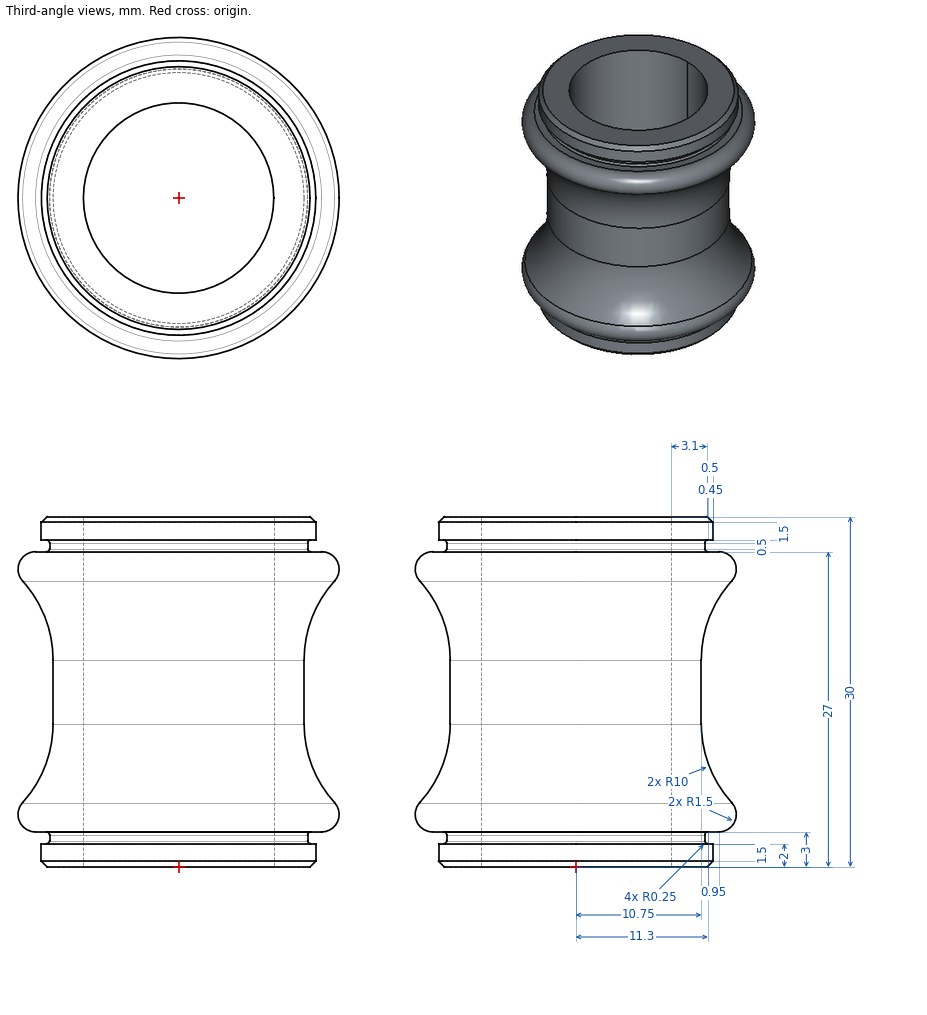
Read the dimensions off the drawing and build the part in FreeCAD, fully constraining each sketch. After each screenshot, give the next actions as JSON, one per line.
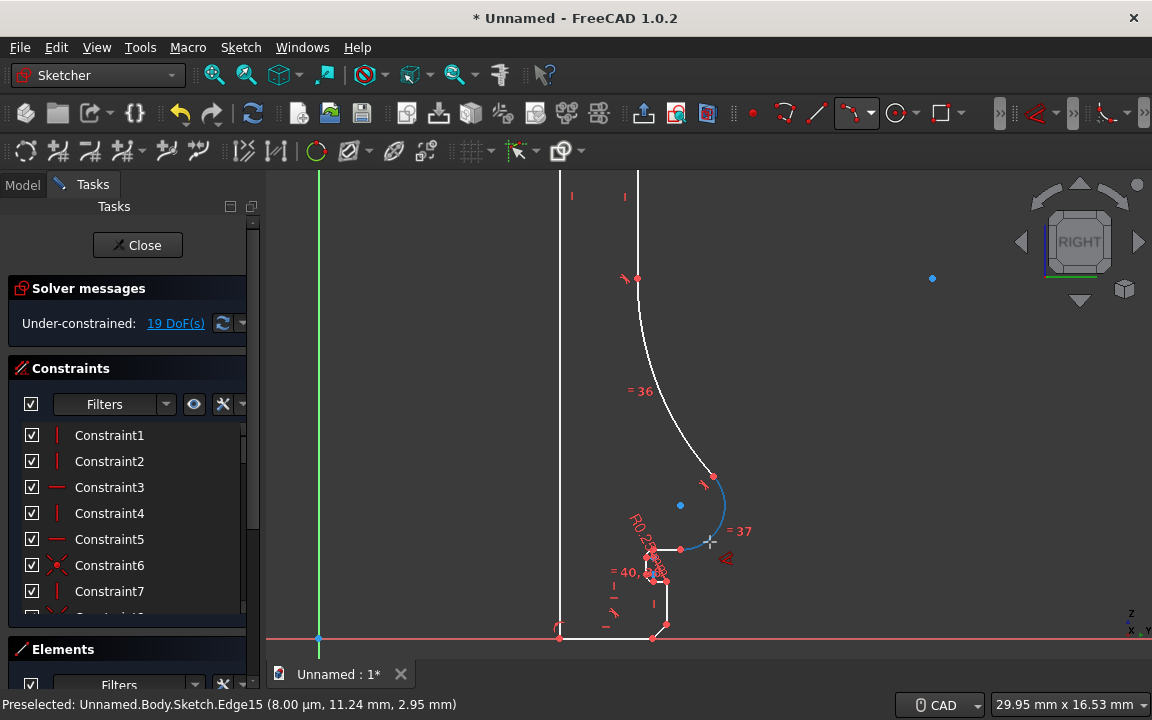
{"action": "left_click", "coordinate": [709, 540]}
{"action": "left_click", "coordinate": [729, 565]}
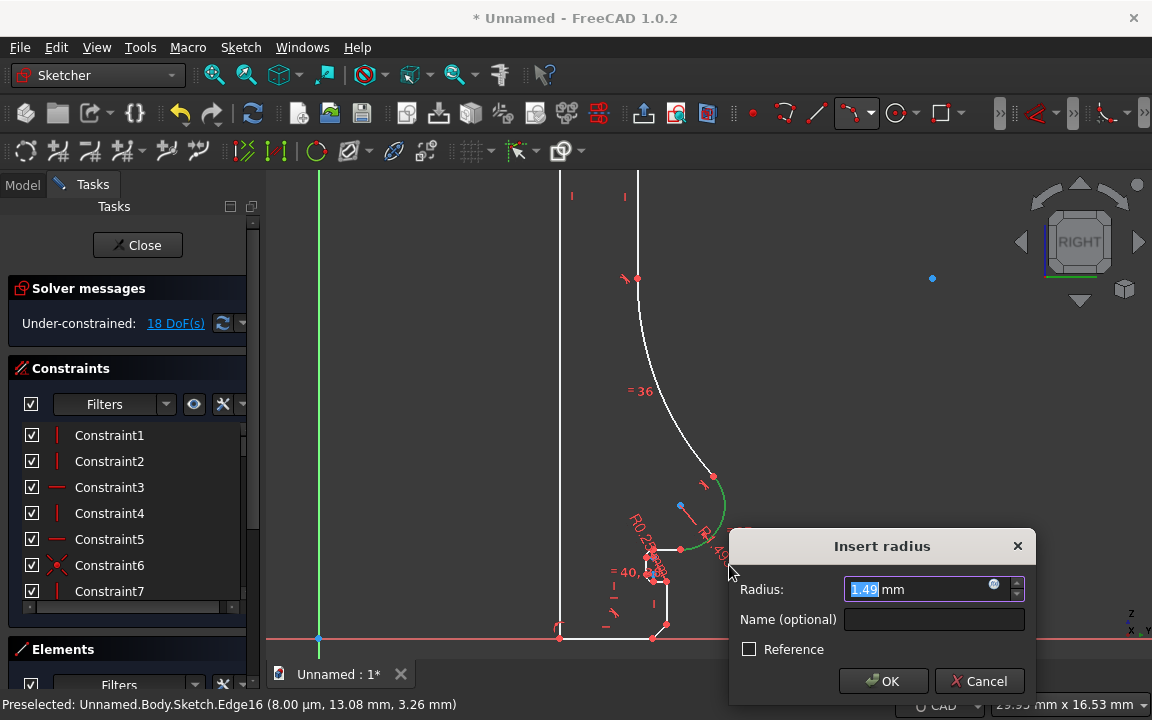
{"action": "type", "text": "1.5"}
{"action": "key", "text": "Return"}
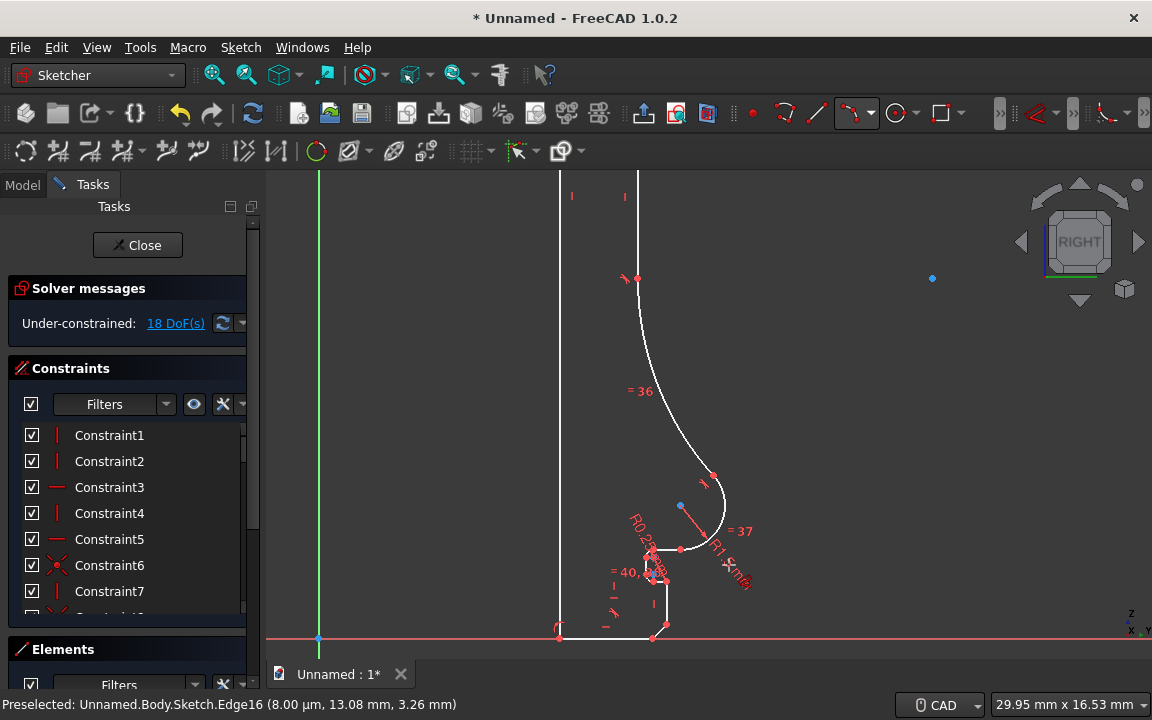
{"action": "left_click", "coordinate": [645, 343]}
{"action": "left_click", "coordinate": [614, 350]}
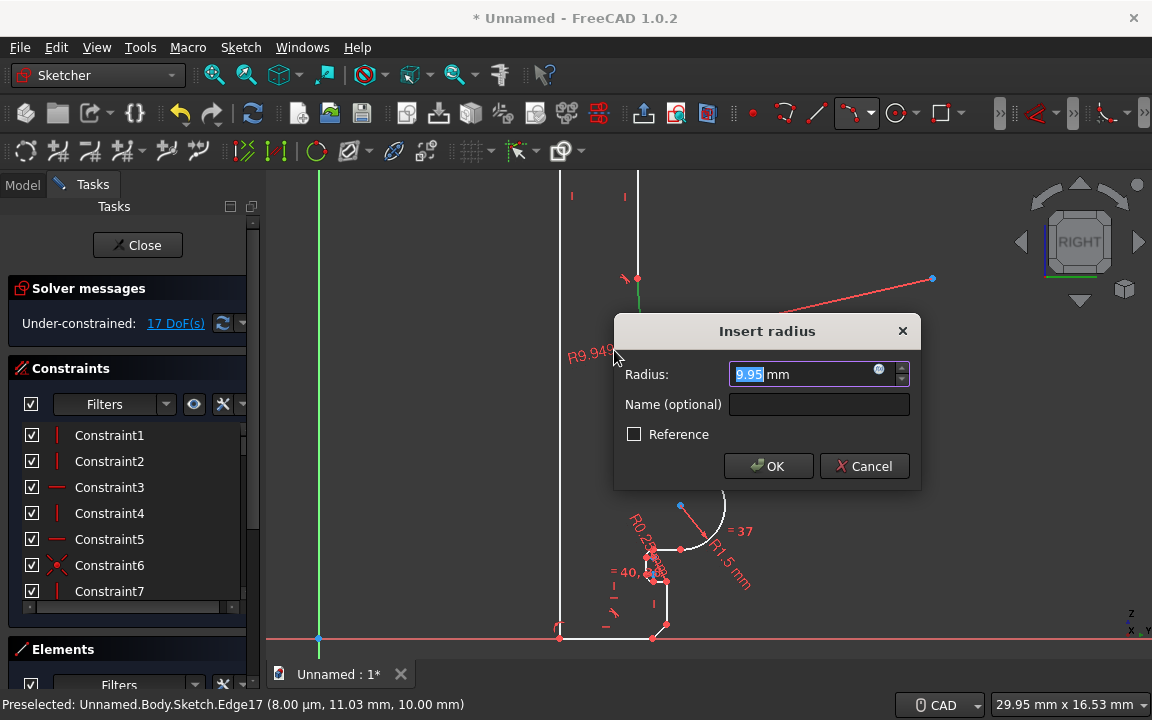
{"action": "type", "text": "10"}
{"action": "key", "text": "Return"}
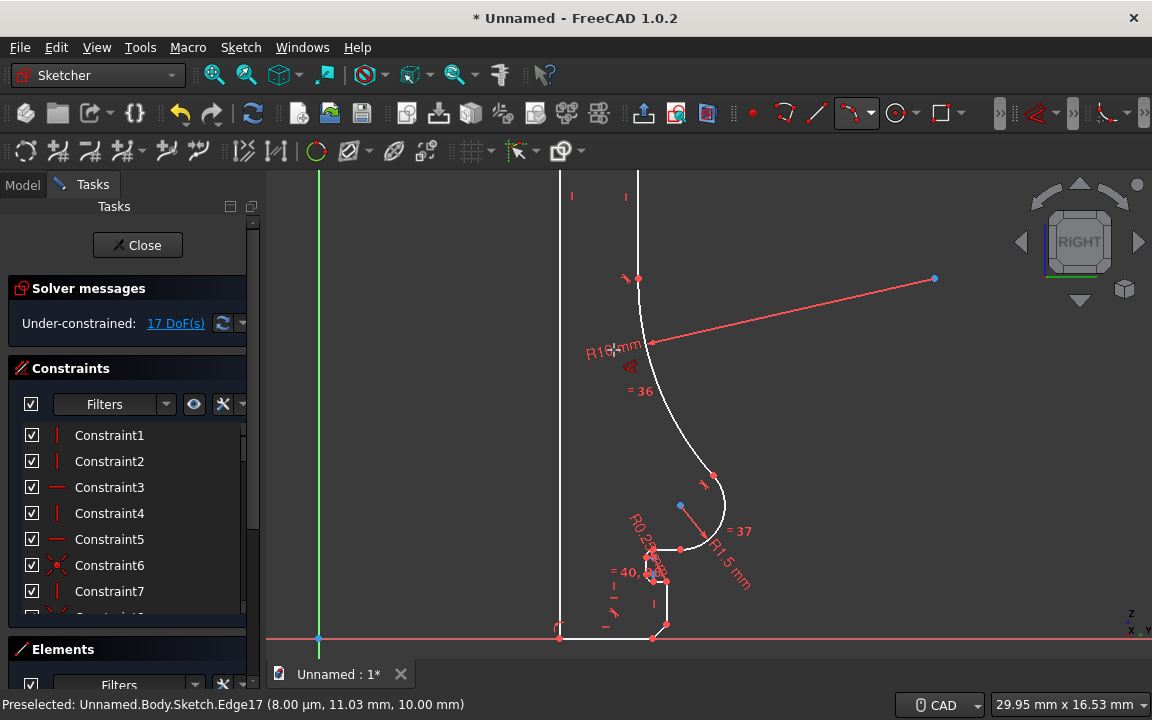
{"action": "left_click", "coordinate": [560, 373]}
{"action": "left_click", "coordinate": [594, 414]}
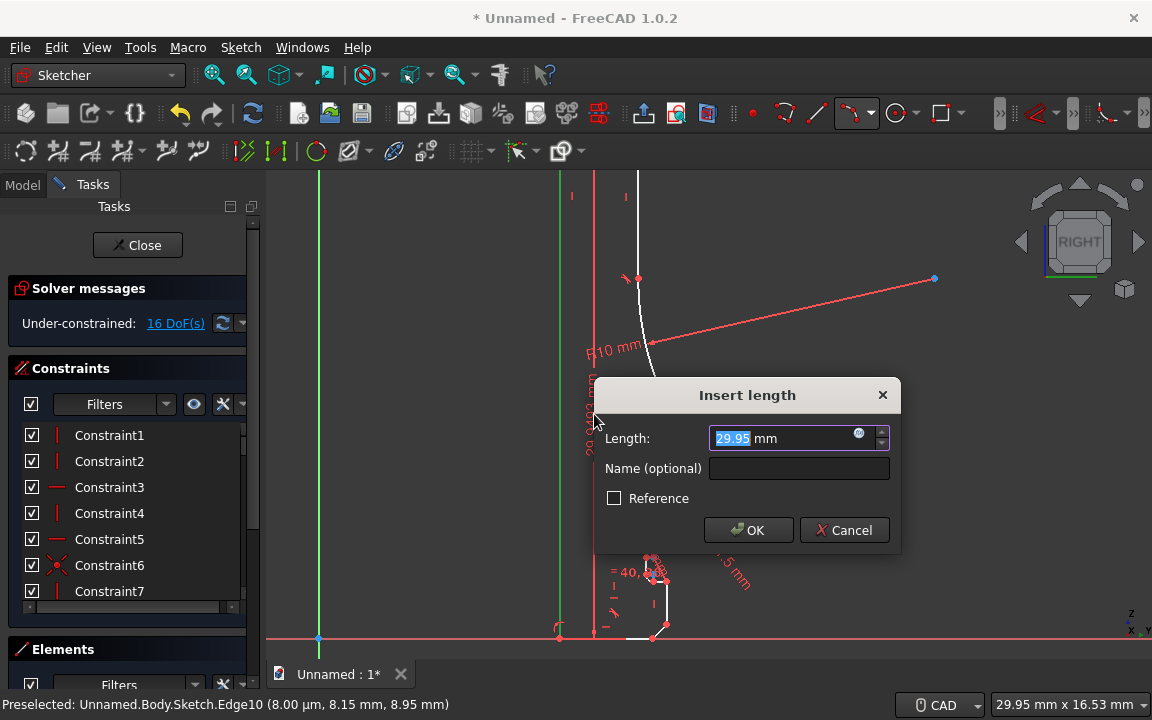
{"action": "type", "text": "30"}
{"action": "key", "text": "Return"}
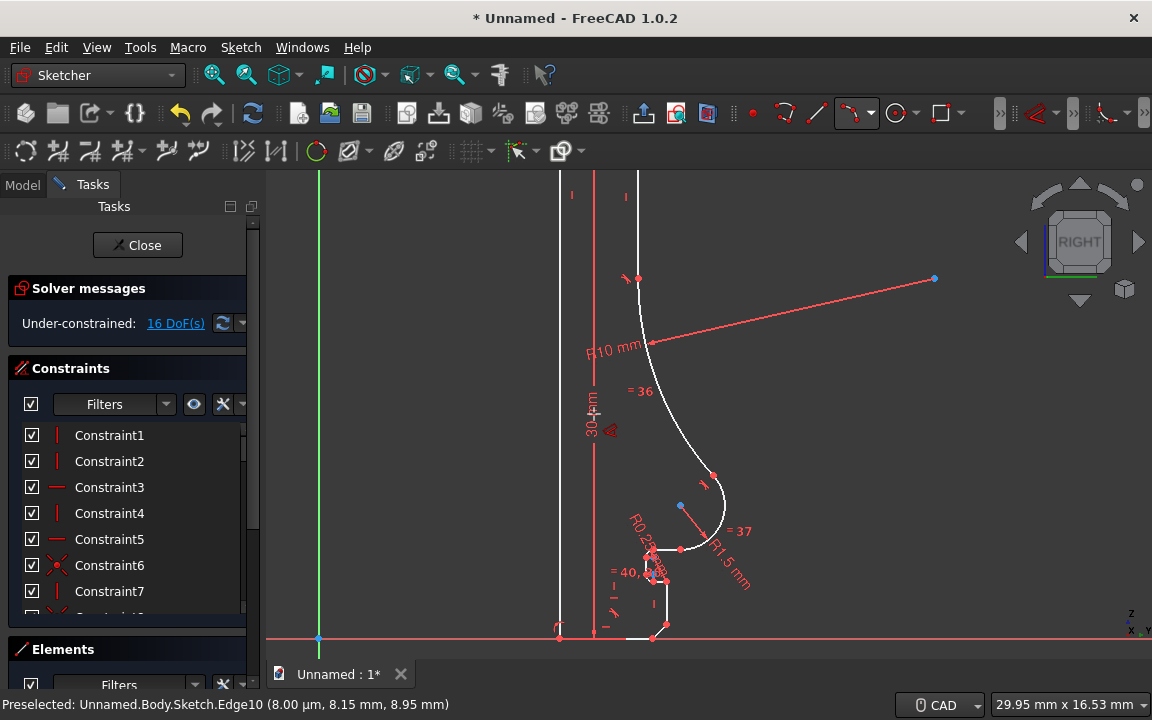
{"action": "scroll", "coordinate": [654, 550], "scroll_direction": "up", "scroll_amount": 3}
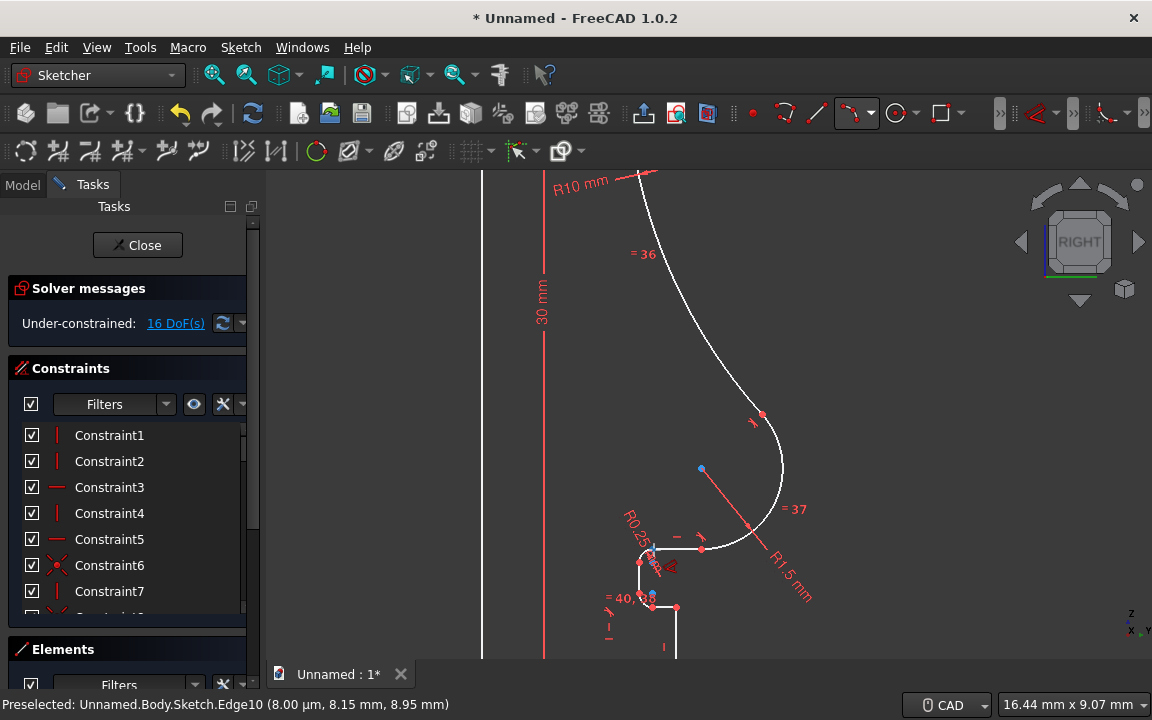
{"action": "left_click", "coordinate": [653, 549]}
{"action": "left_click", "coordinate": [687, 590]}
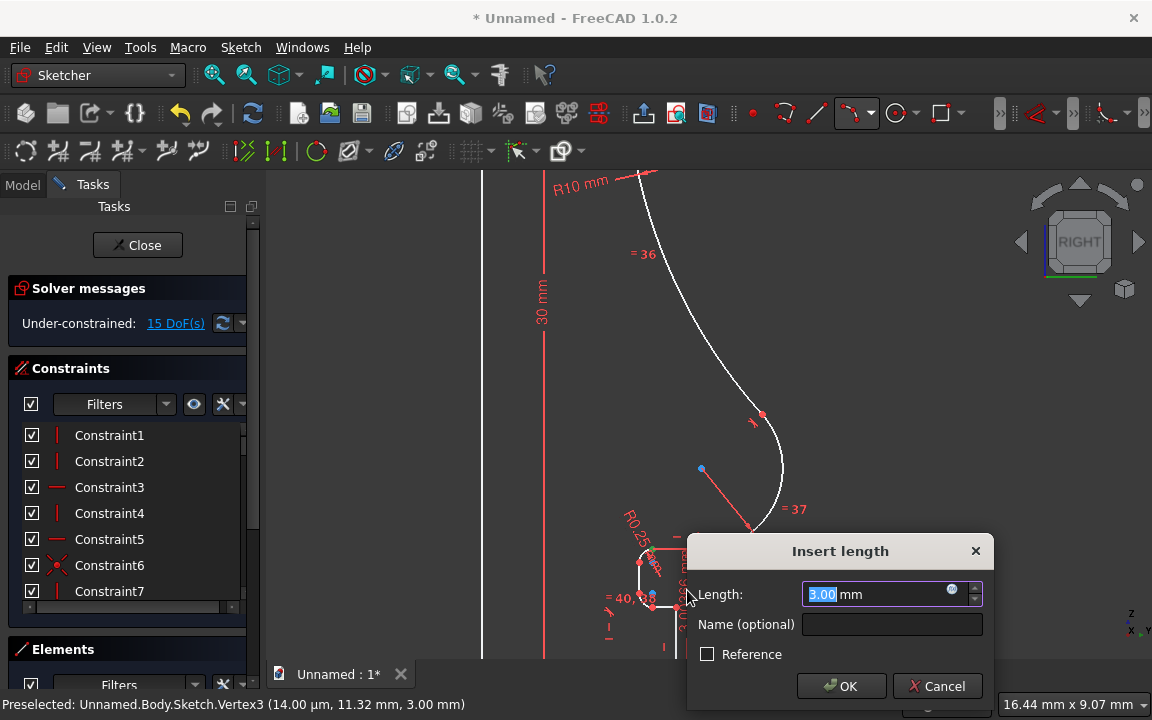
{"action": "type", "text": "3"}
{"action": "key", "text": "Return"}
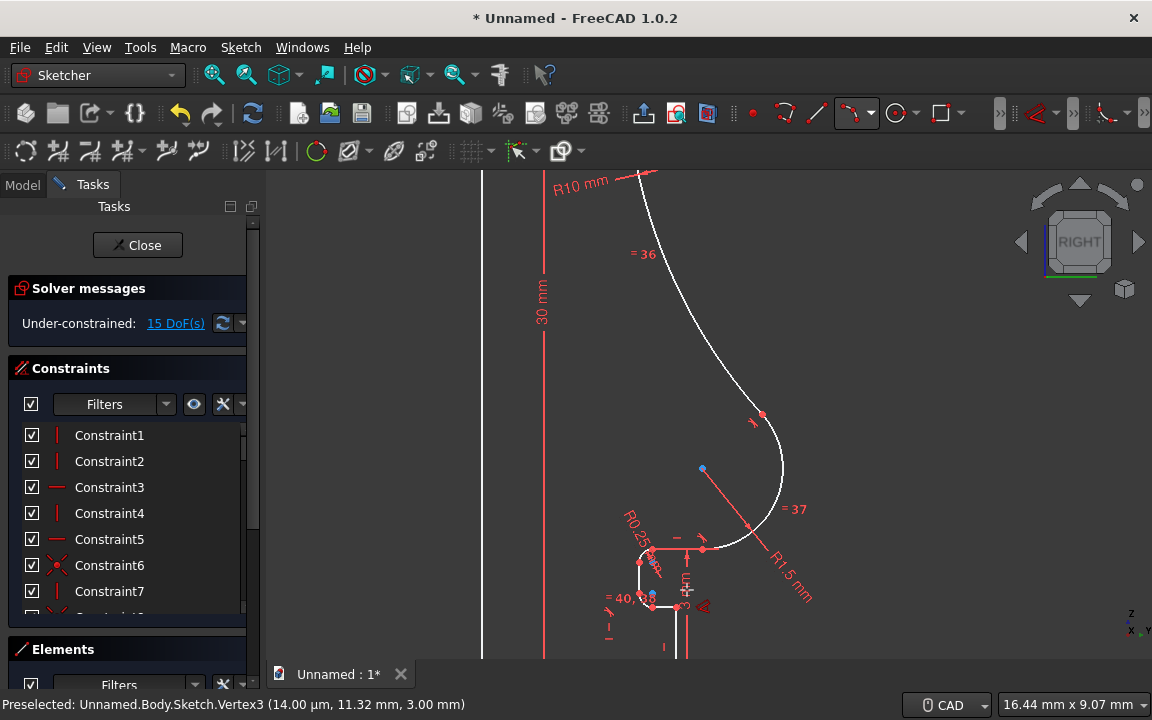
{"action": "left_click", "coordinate": [676, 607]}
{"action": "left_click", "coordinate": [710, 619]}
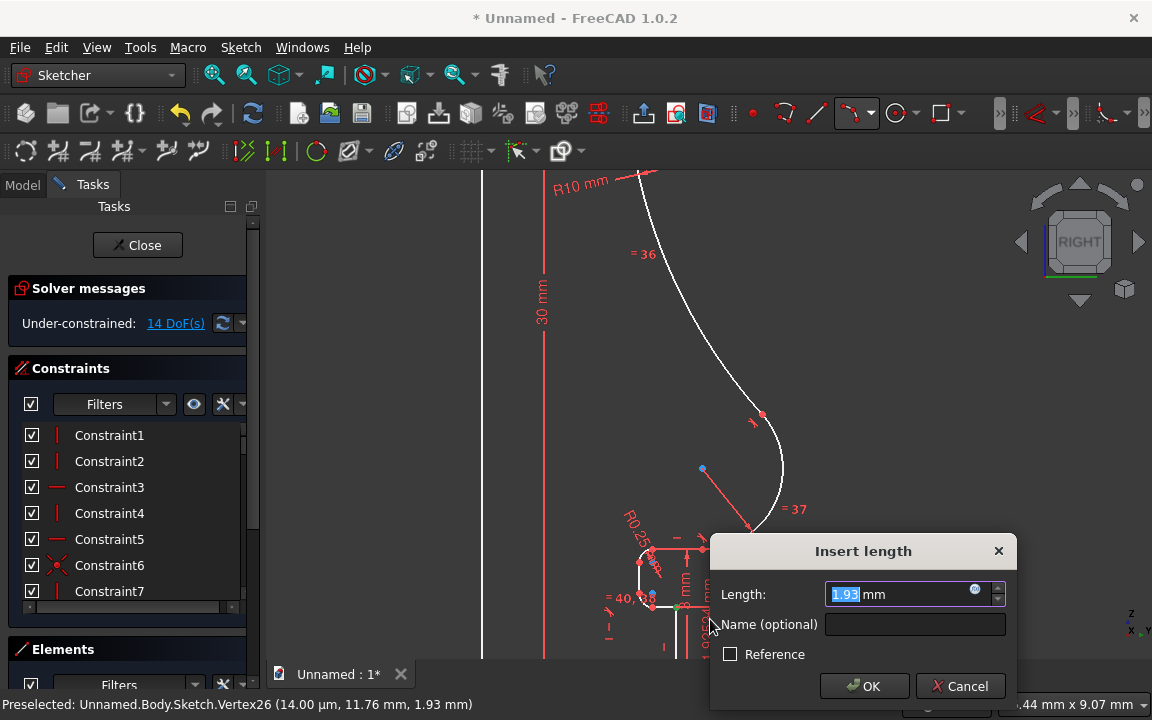
{"action": "type", "text": "2"}
{"action": "key", "text": "Return"}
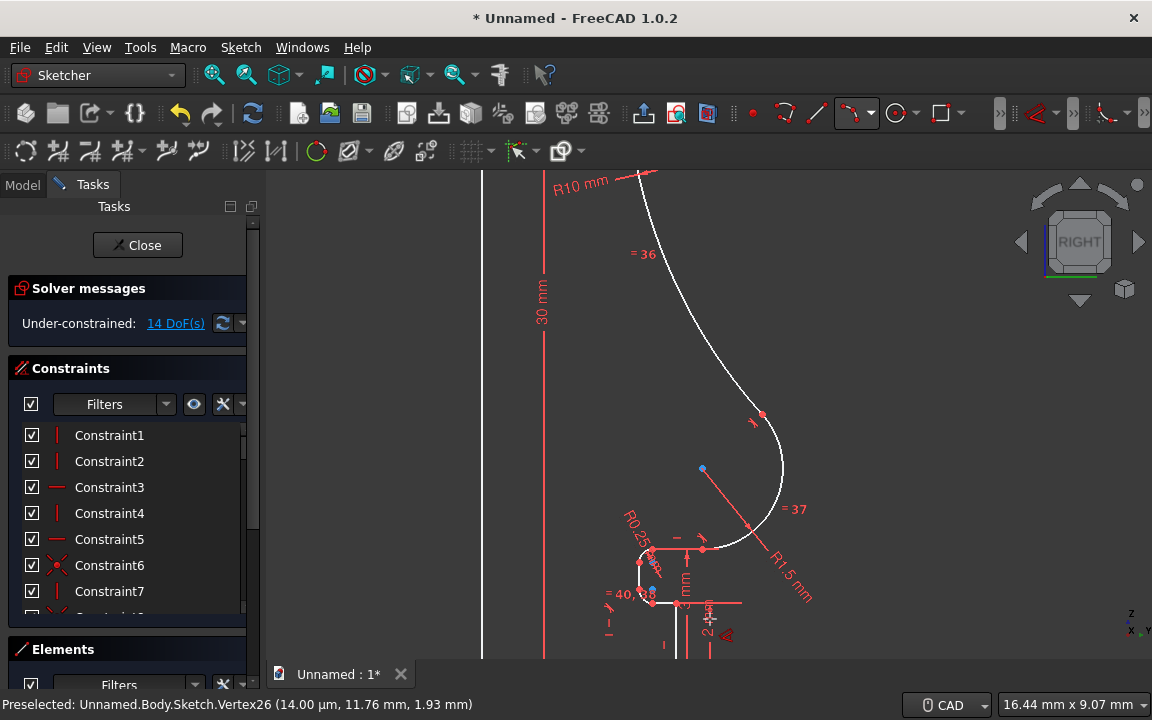
{"action": "scroll", "coordinate": [699, 544], "scroll_direction": "down", "scroll_amount": 8}